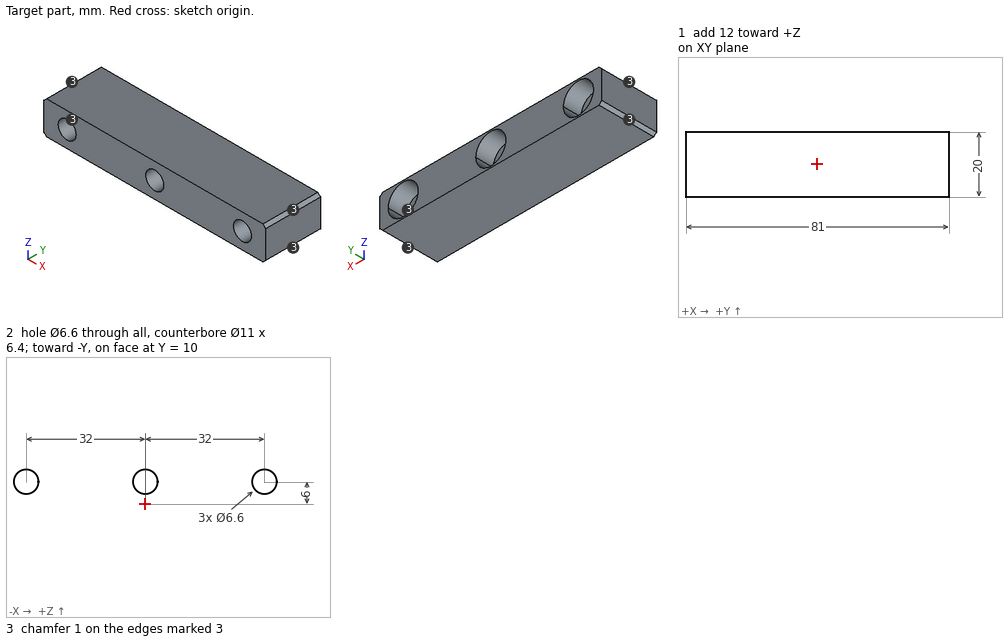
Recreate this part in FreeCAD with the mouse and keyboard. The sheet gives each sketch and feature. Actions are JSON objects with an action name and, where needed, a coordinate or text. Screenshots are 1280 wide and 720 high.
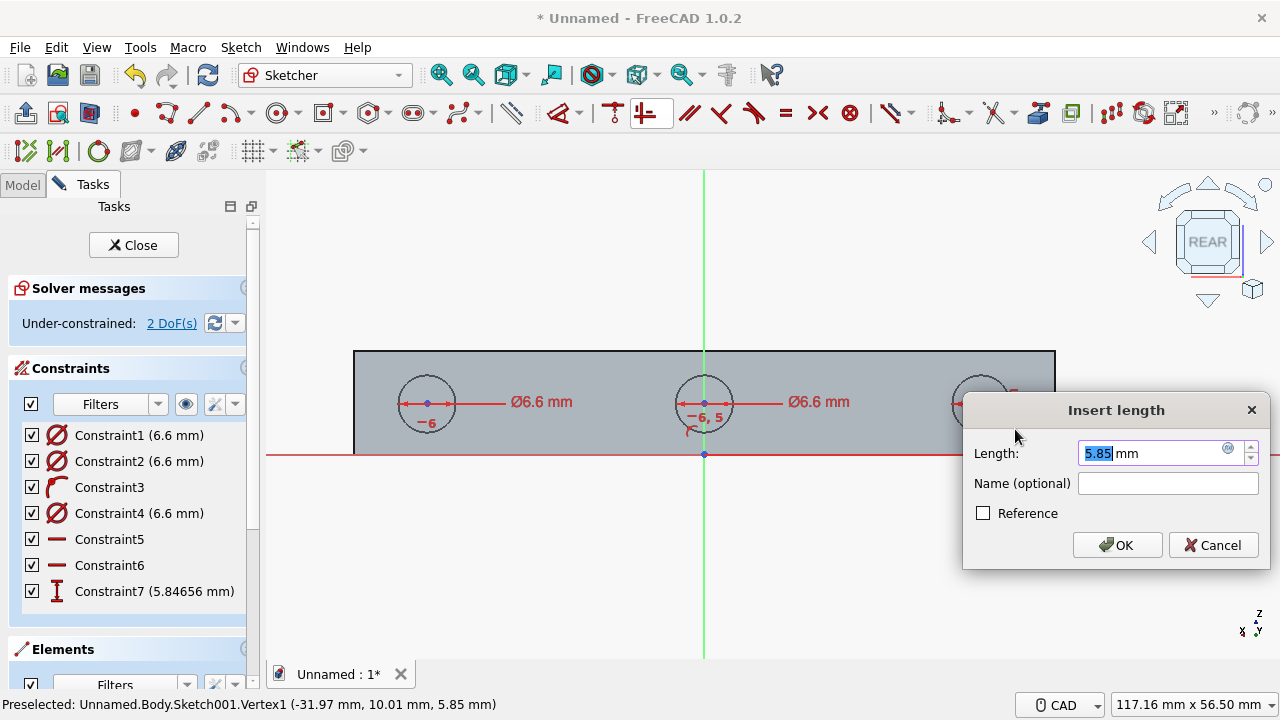
{"action": "type", "text": "6"}
{"action": "key", "text": "Return"}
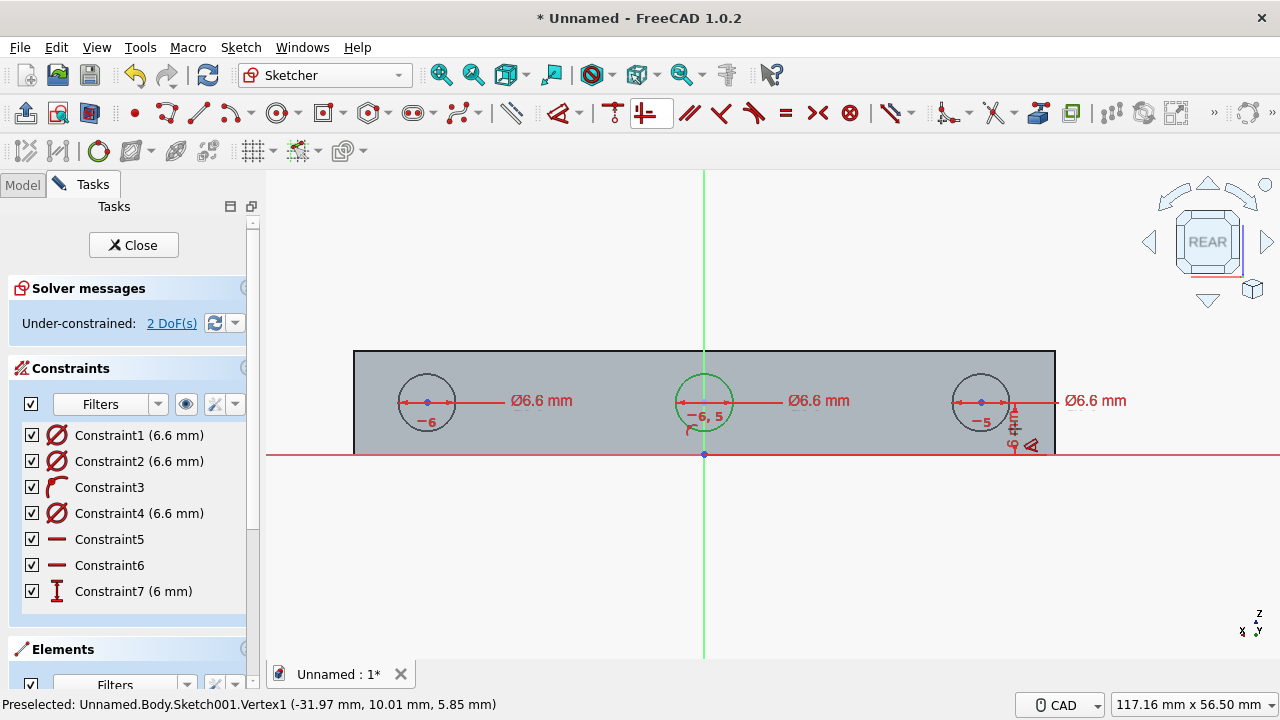
{"action": "left_click", "coordinate": [981, 403]}
{"action": "left_click", "coordinate": [843, 489]}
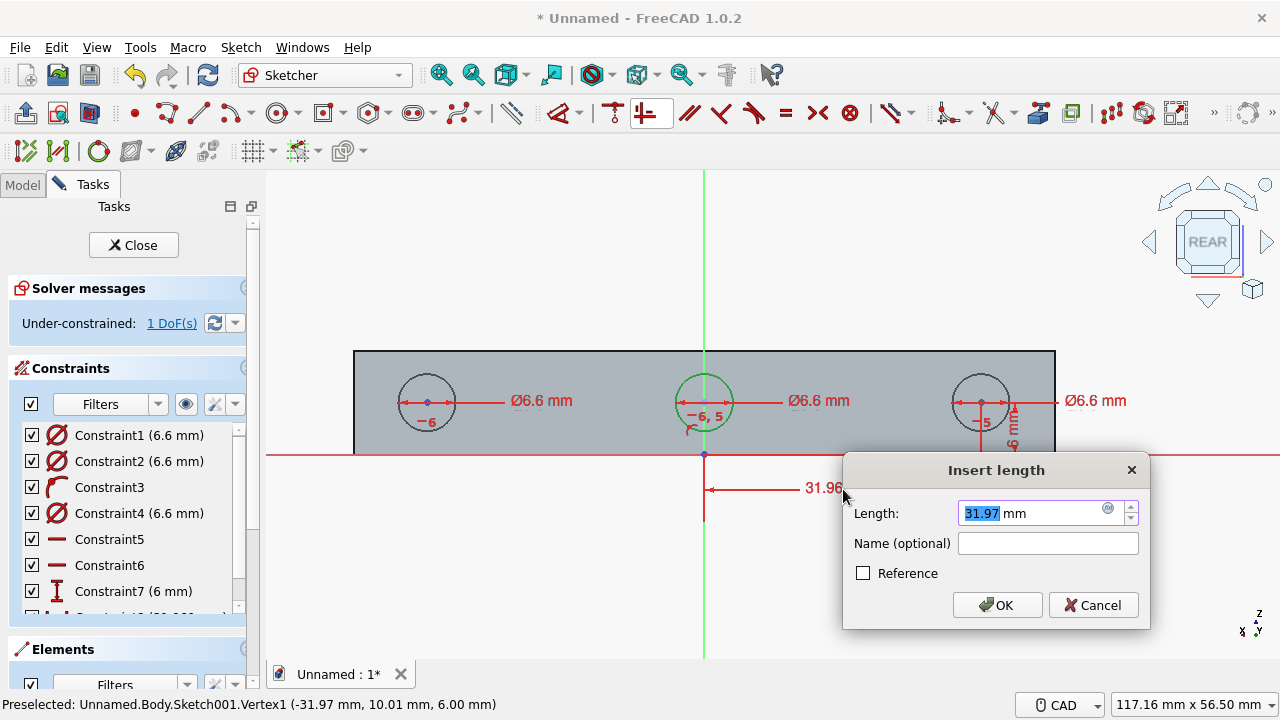
{"action": "type", "text": "32"}
{"action": "key", "text": "Return"}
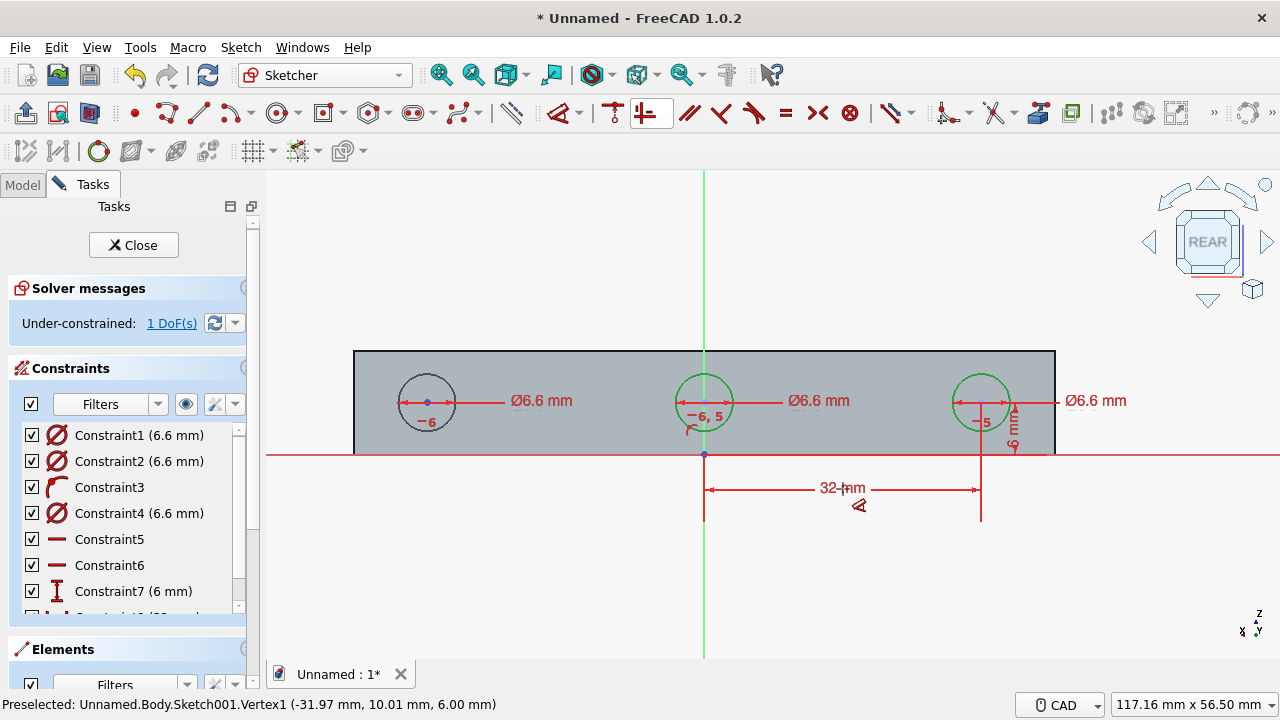
{"action": "left_click", "coordinate": [427, 403]}
{"action": "left_click", "coordinate": [566, 489]}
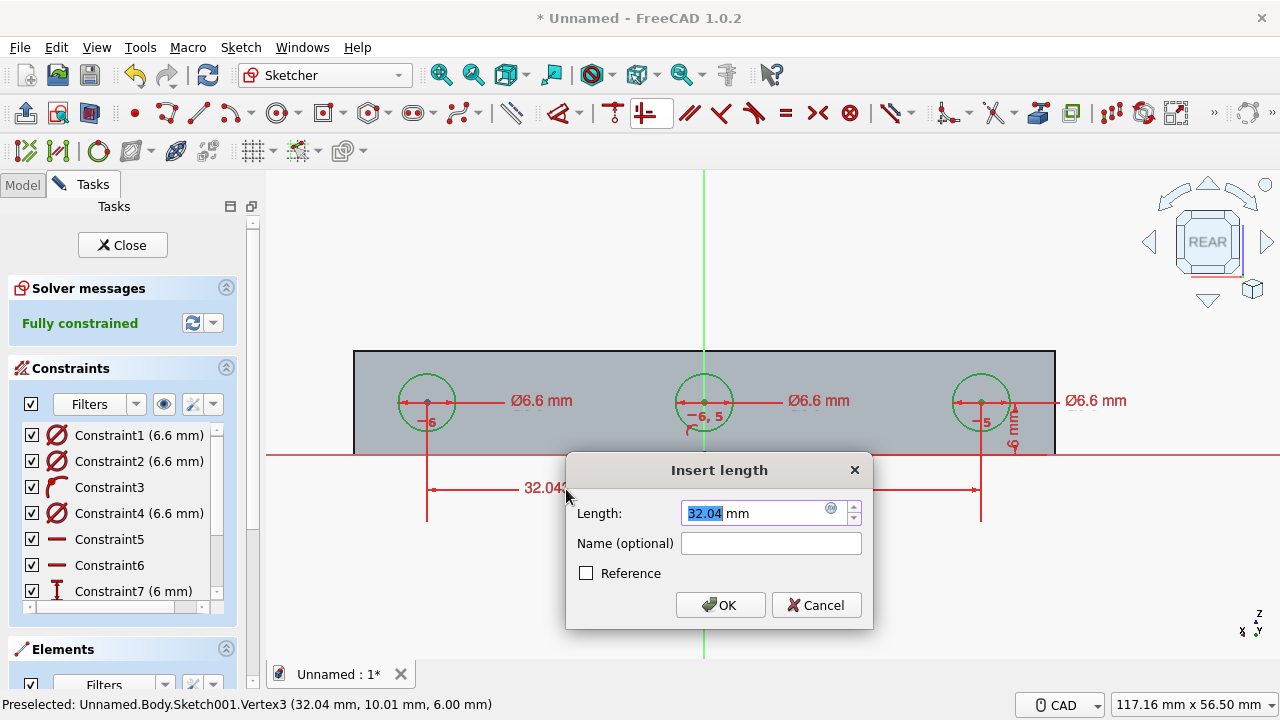
{"action": "type", "text": "32"}
{"action": "key", "text": "Return"}
{"action": "key", "text": "Escape"}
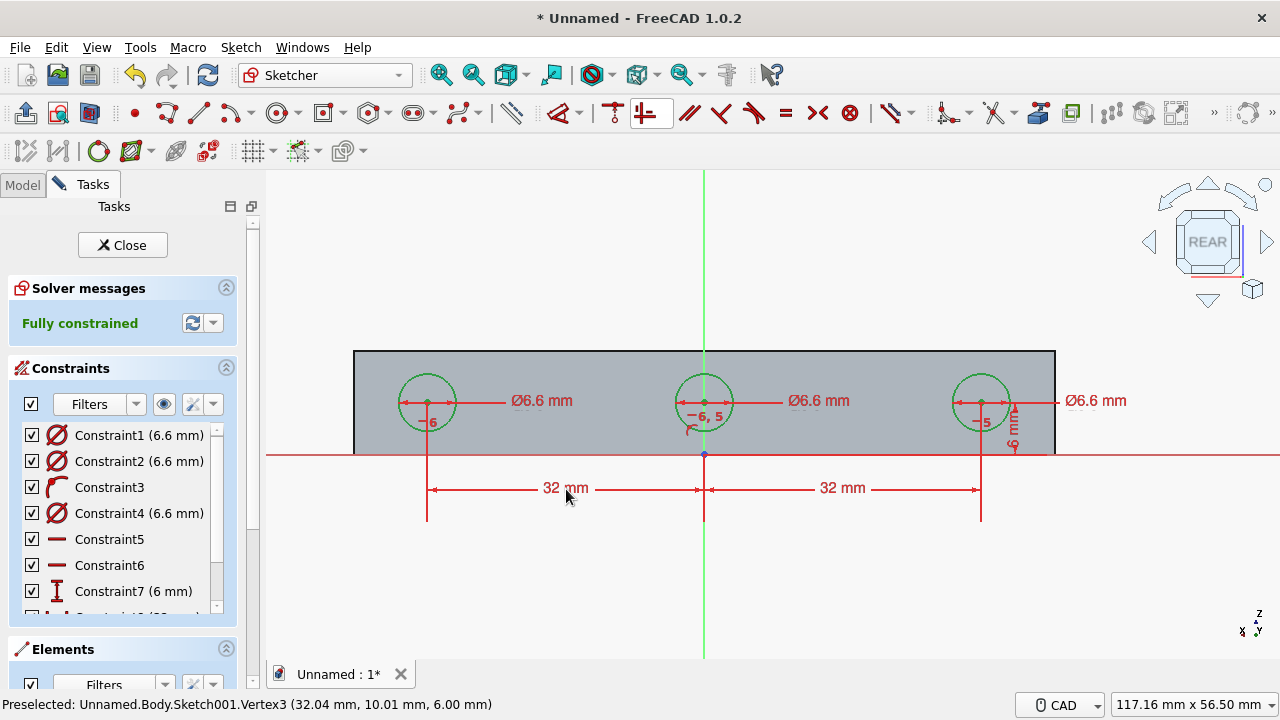
{"action": "left_click", "coordinate": [123, 245]}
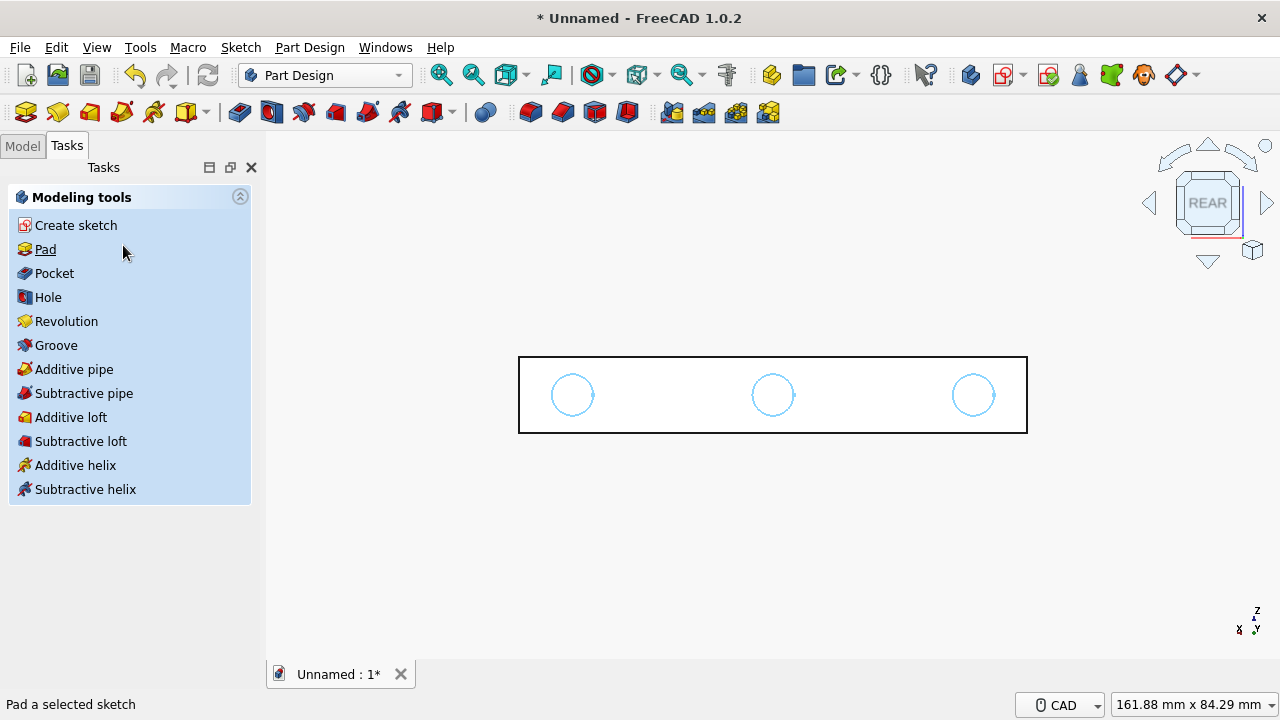
{"action": "left_click", "coordinate": [272, 112]}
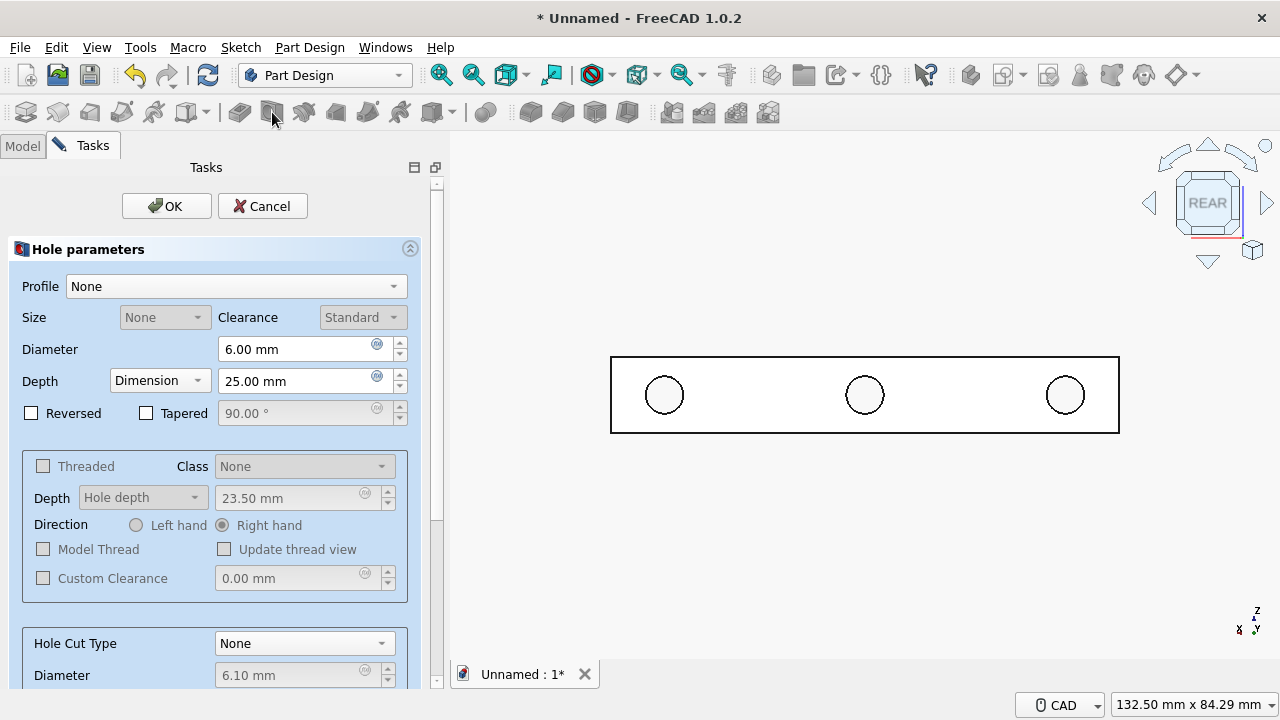
{"action": "triple_click", "coordinate": [305, 349]}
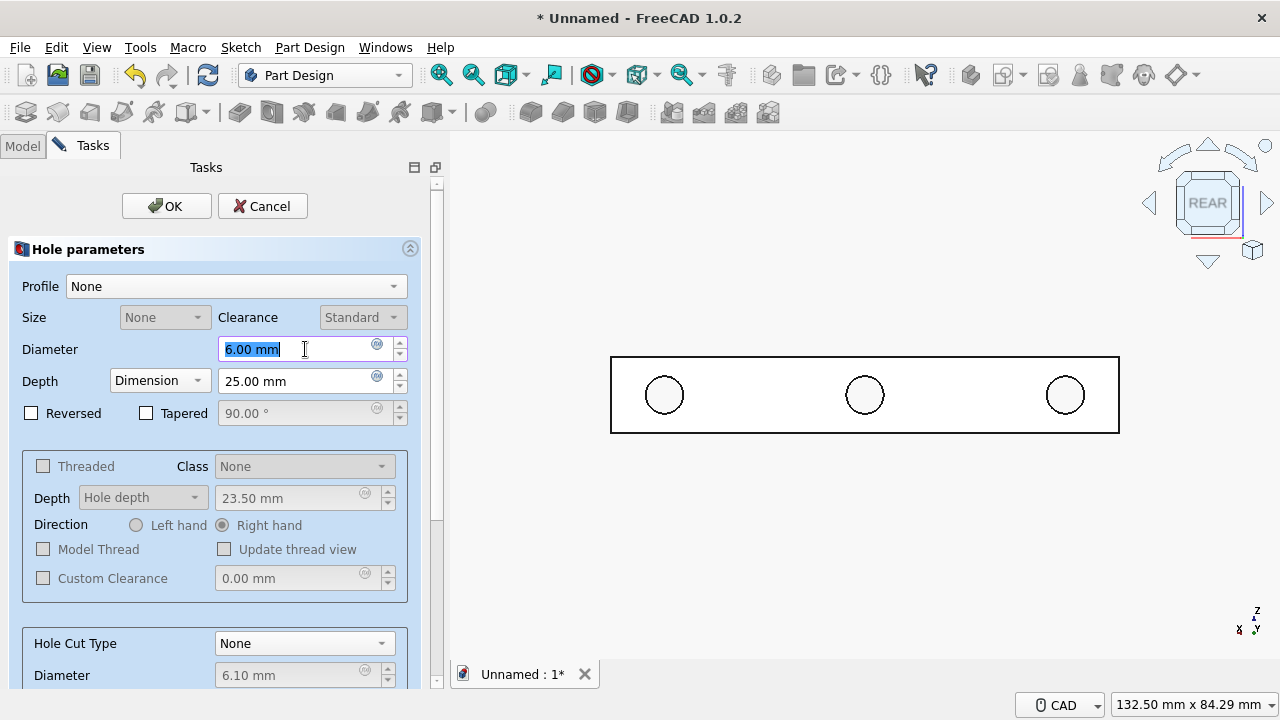
{"action": "type", "text": "6.6"}
{"action": "key", "text": "Tab"}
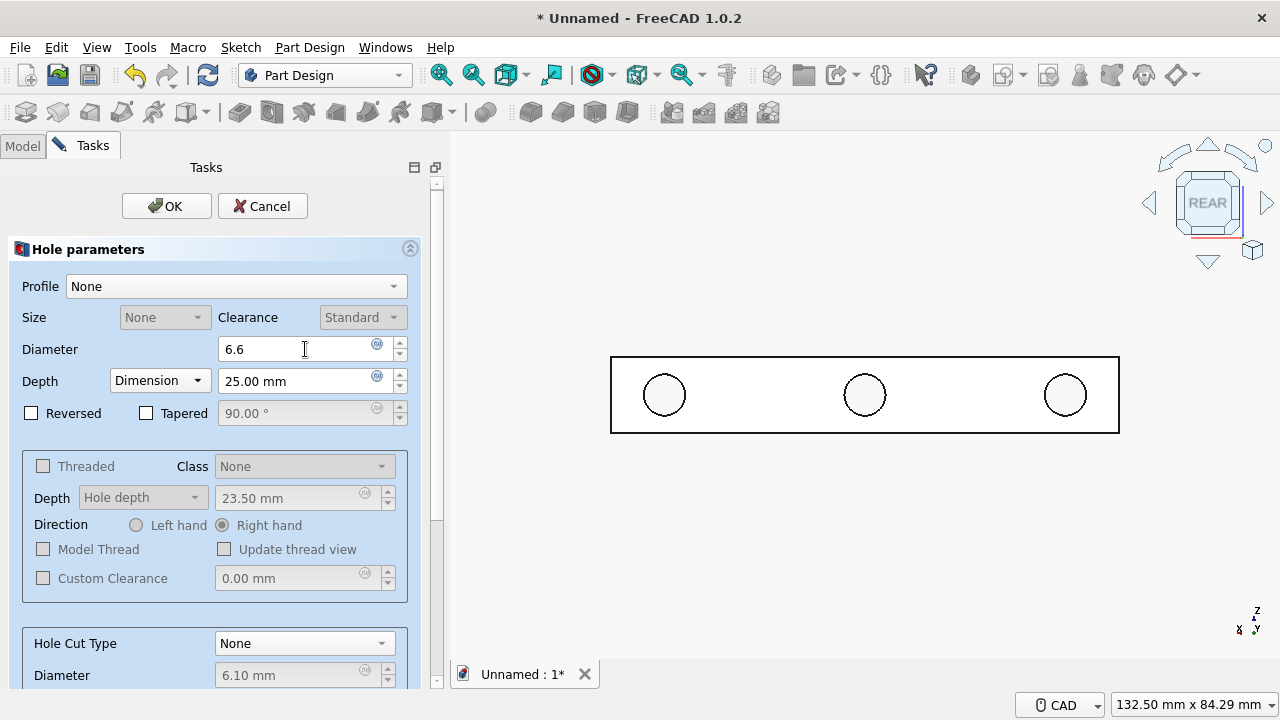
{"action": "left_click", "coordinate": [161, 380]}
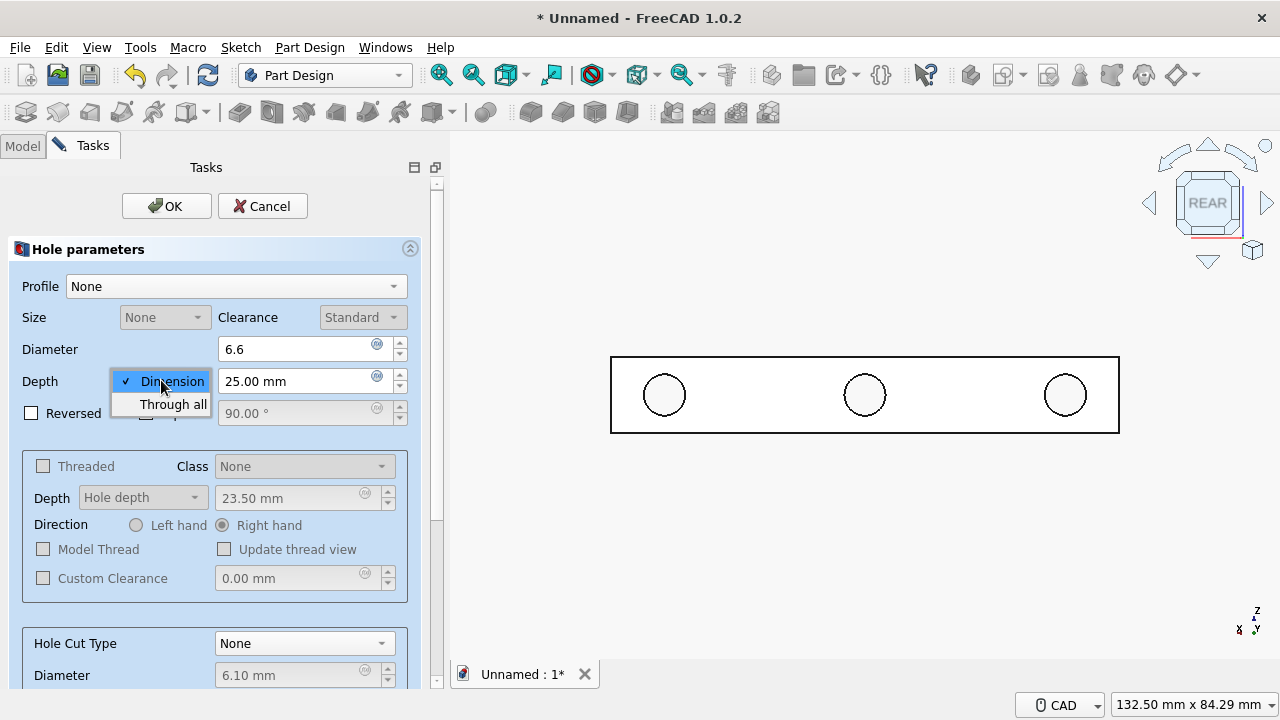
{"action": "left_click", "coordinate": [160, 404]}